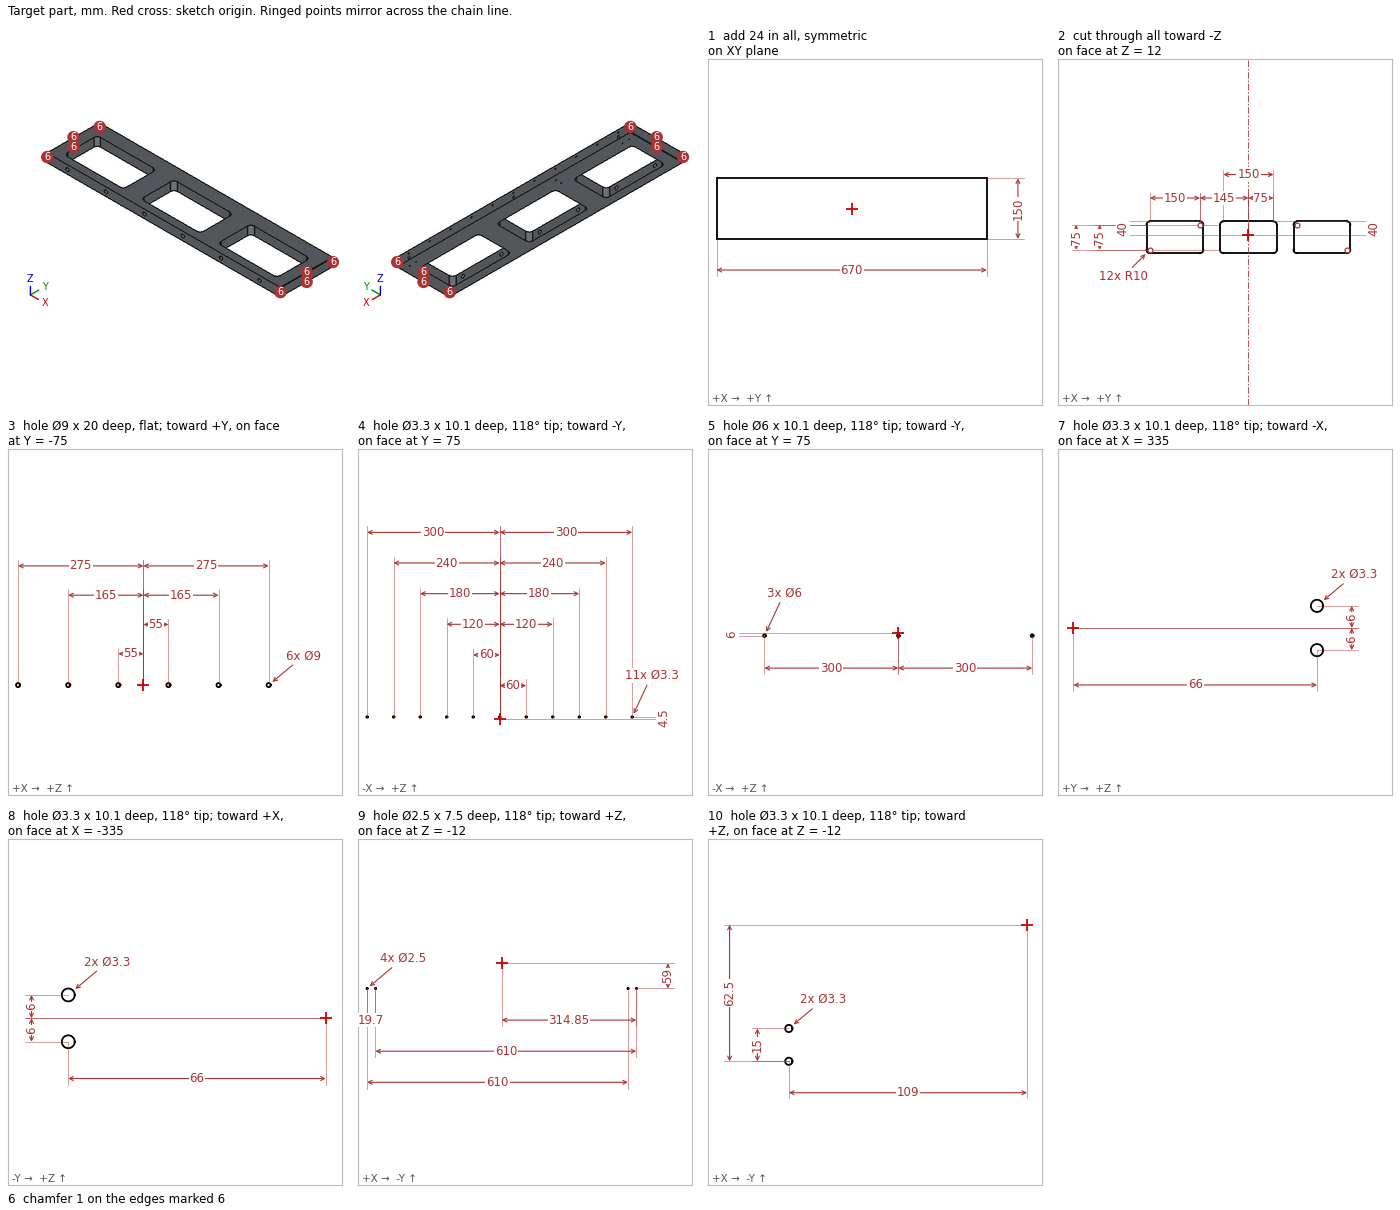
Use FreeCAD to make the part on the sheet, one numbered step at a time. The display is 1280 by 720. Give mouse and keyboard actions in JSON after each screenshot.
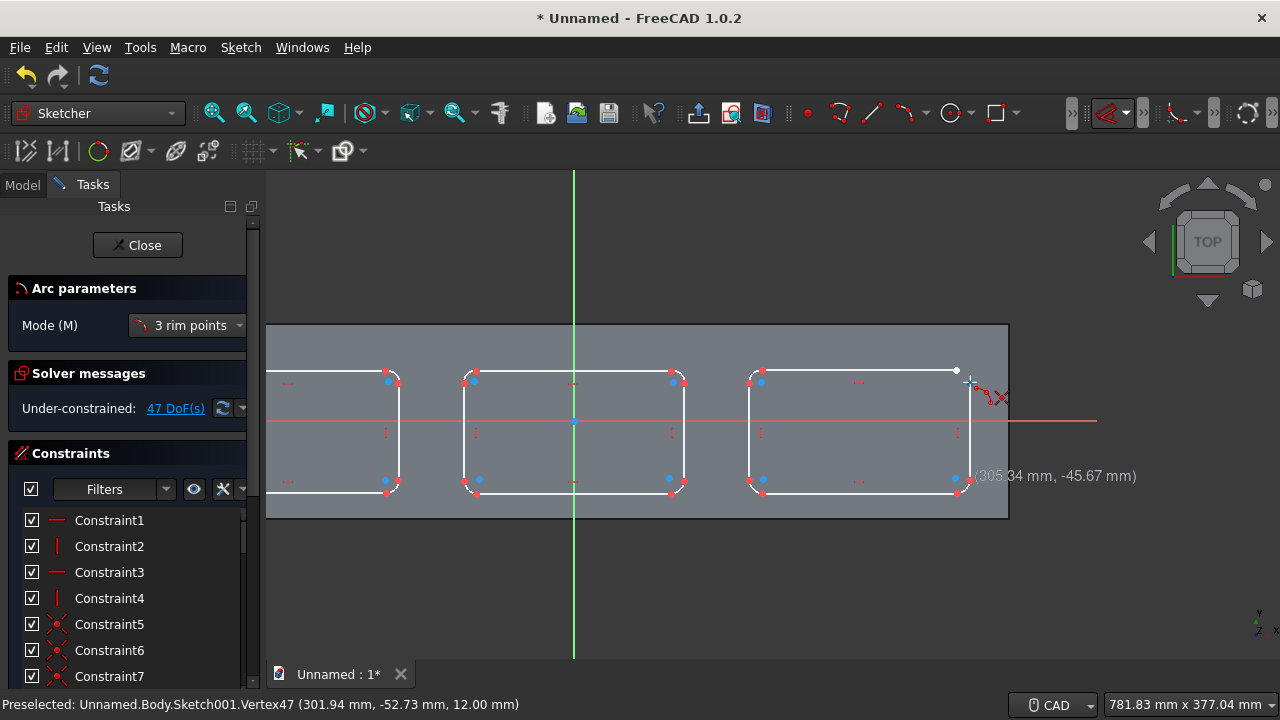
{"action": "left_click", "coordinate": [970, 384]}
{"action": "left_click", "coordinate": [956, 370]}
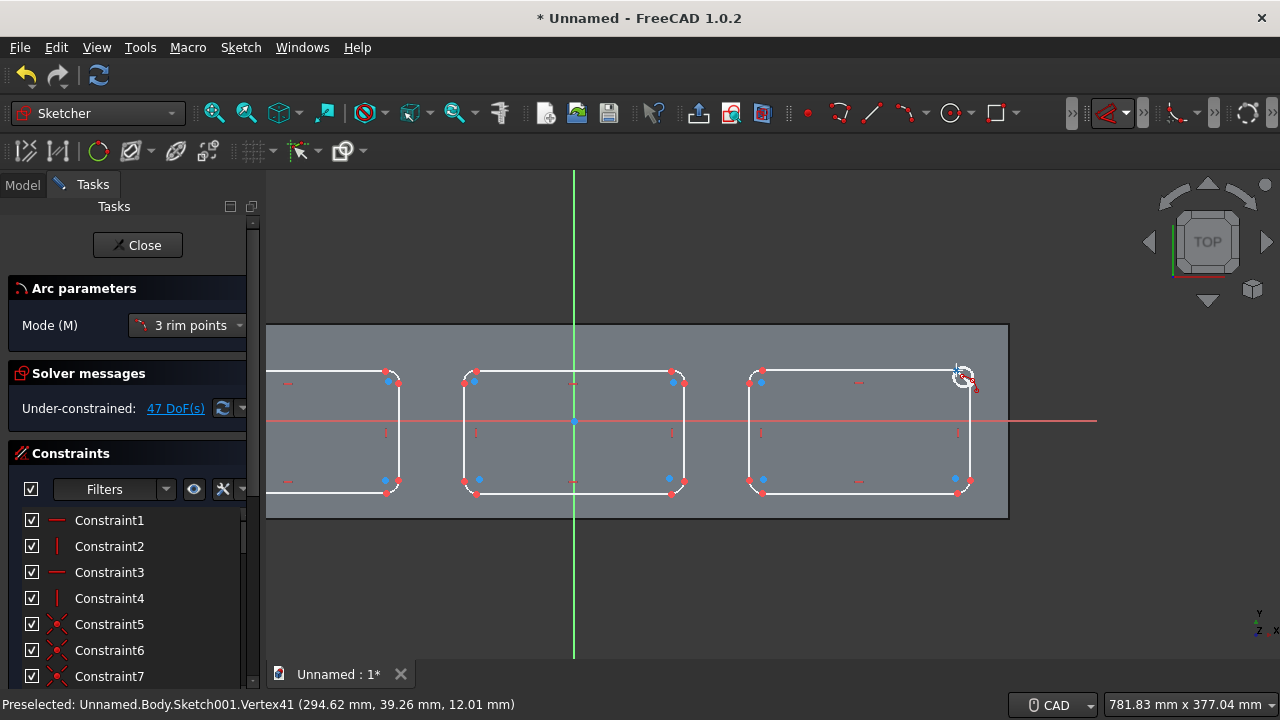
{"action": "scroll", "coordinate": [966, 373], "scroll_direction": "up", "scroll_amount": 8}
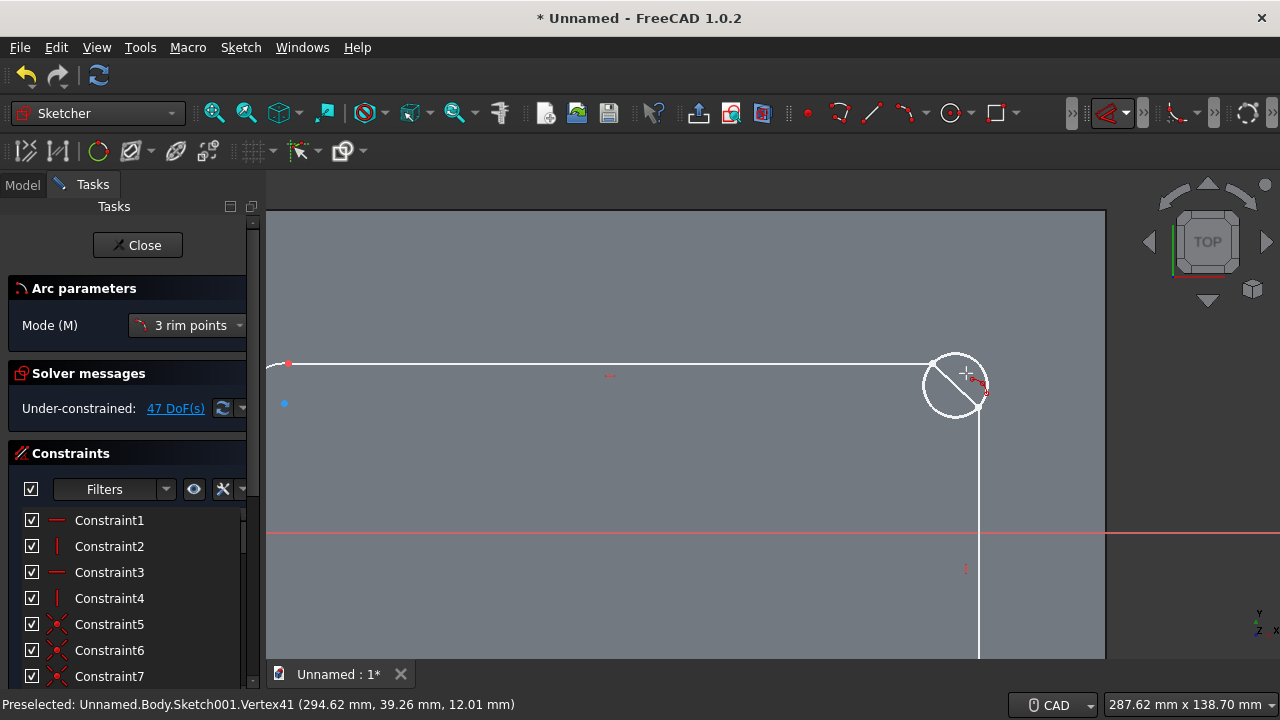
{"action": "left_click", "coordinate": [963, 373]}
{"action": "key", "text": "Escape"}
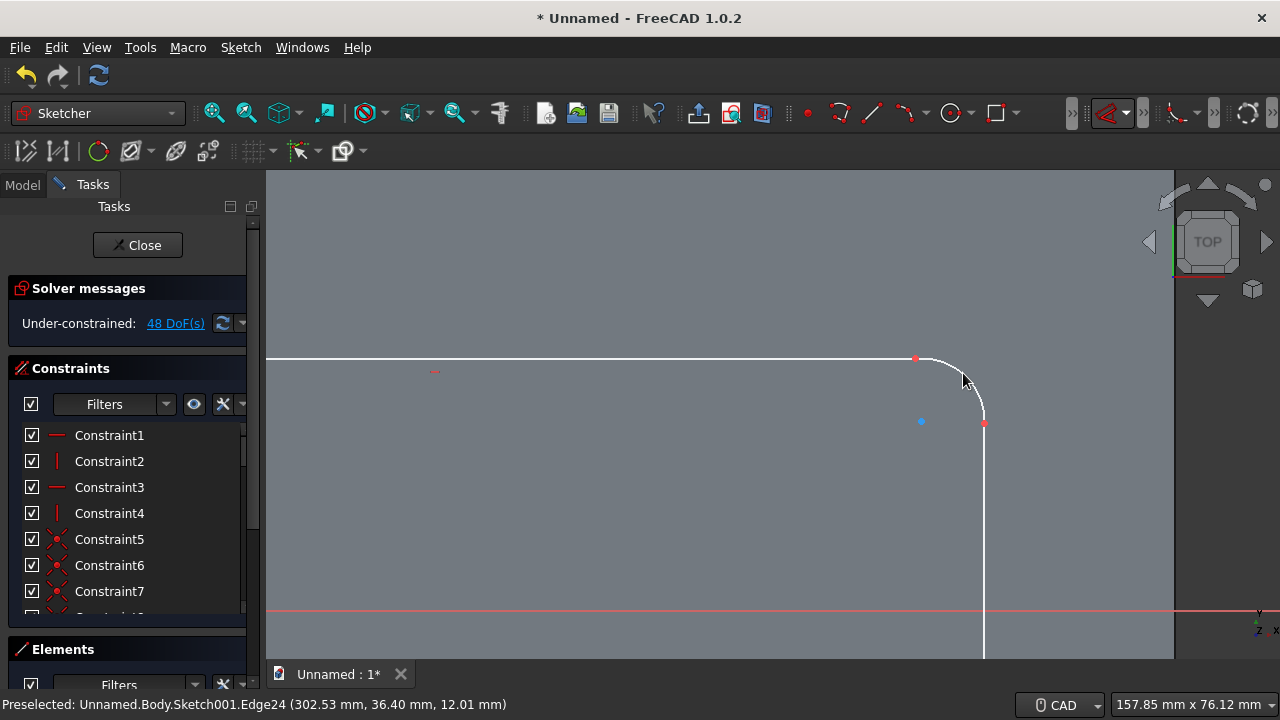
{"action": "scroll", "coordinate": [968, 376], "scroll_direction": "down", "scroll_amount": 10}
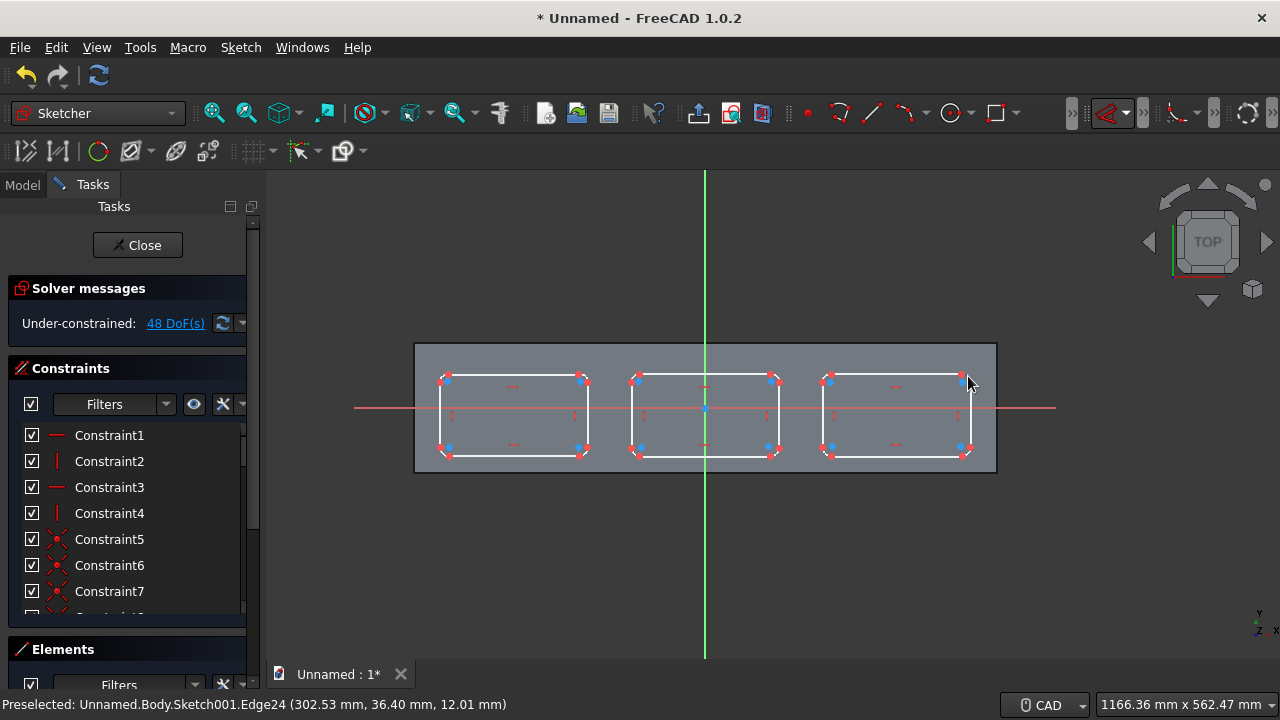
{"action": "left_click", "coordinate": [540, 375]}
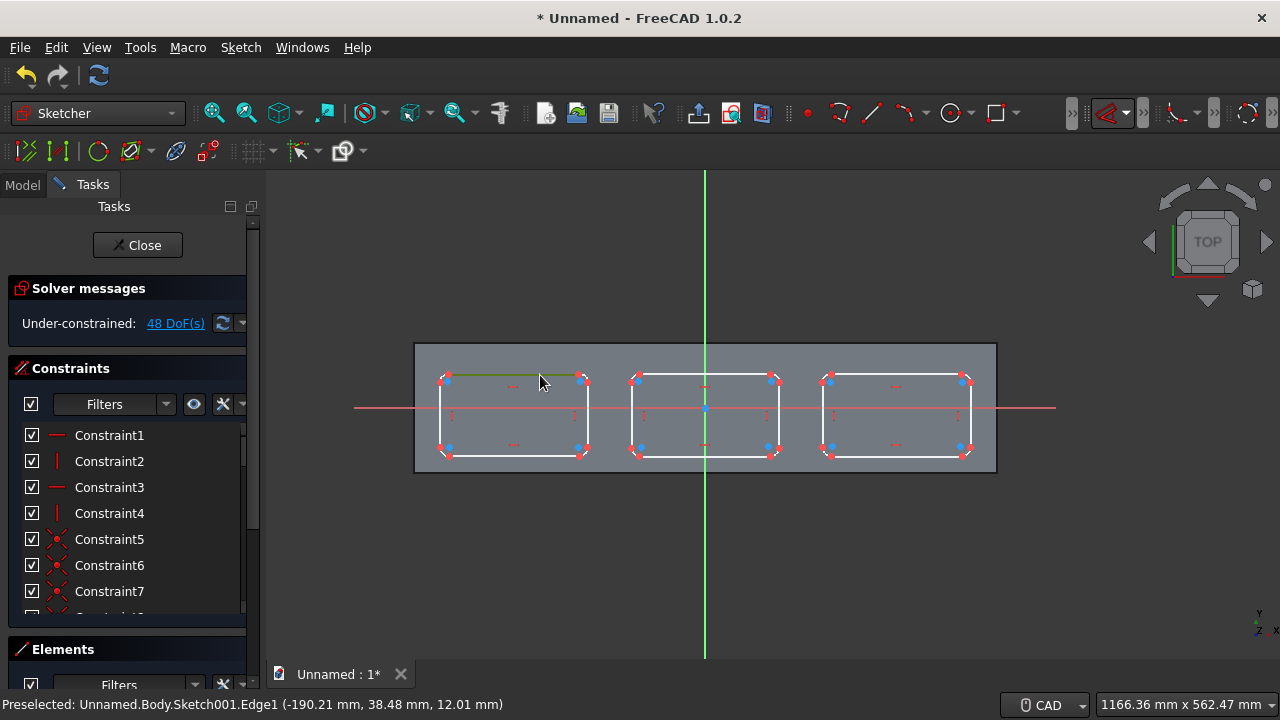
{"action": "scroll", "coordinate": [442, 377], "scroll_direction": "up", "scroll_amount": 4}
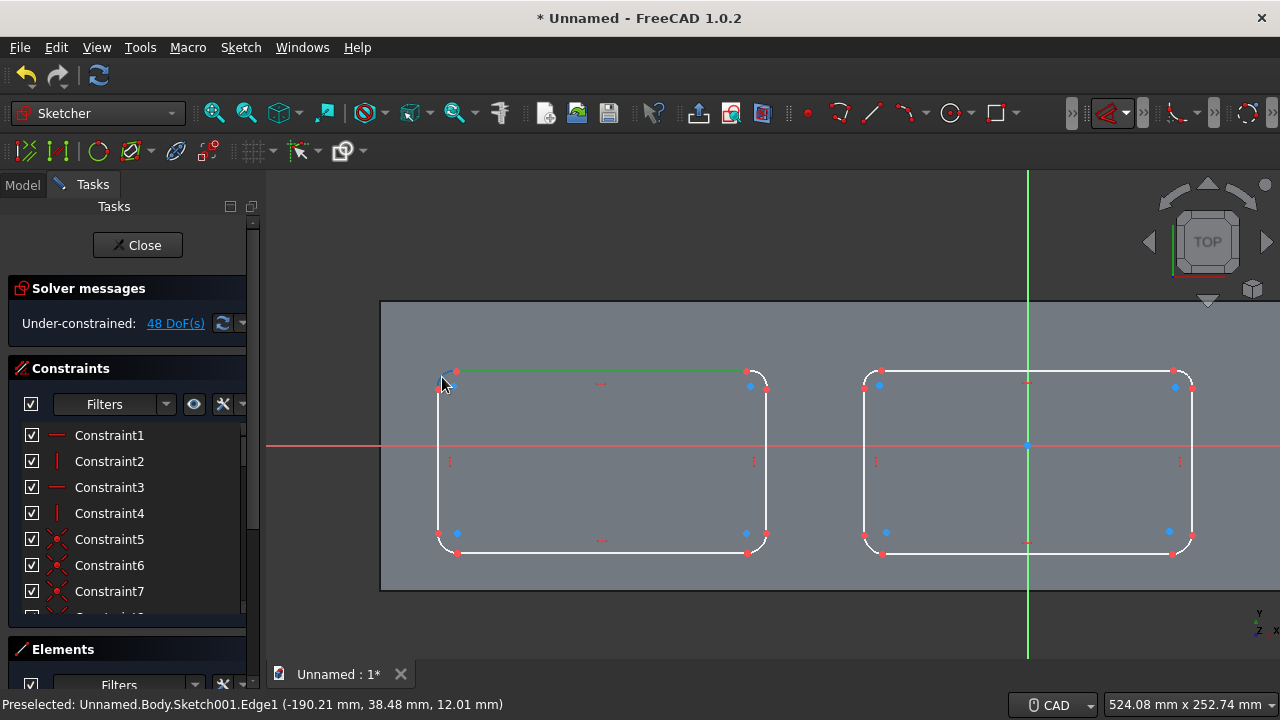
{"action": "left_click", "coordinate": [442, 375]}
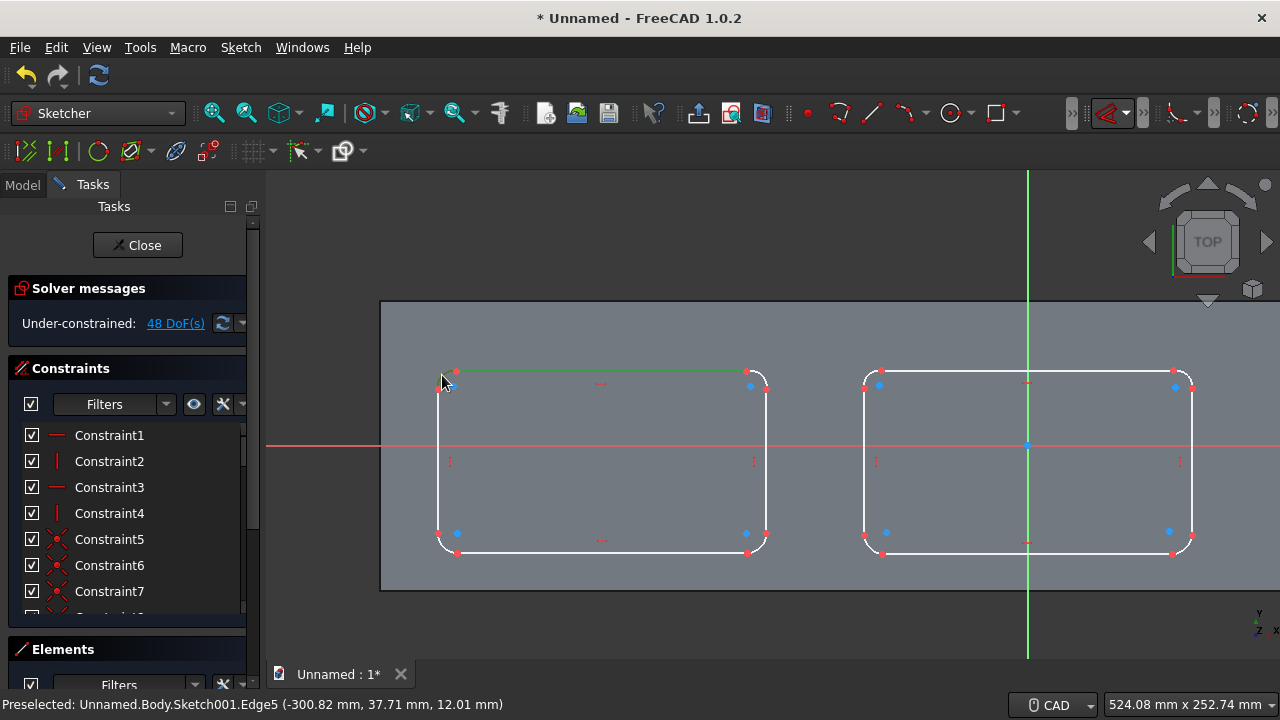
{"action": "key", "text": "t"}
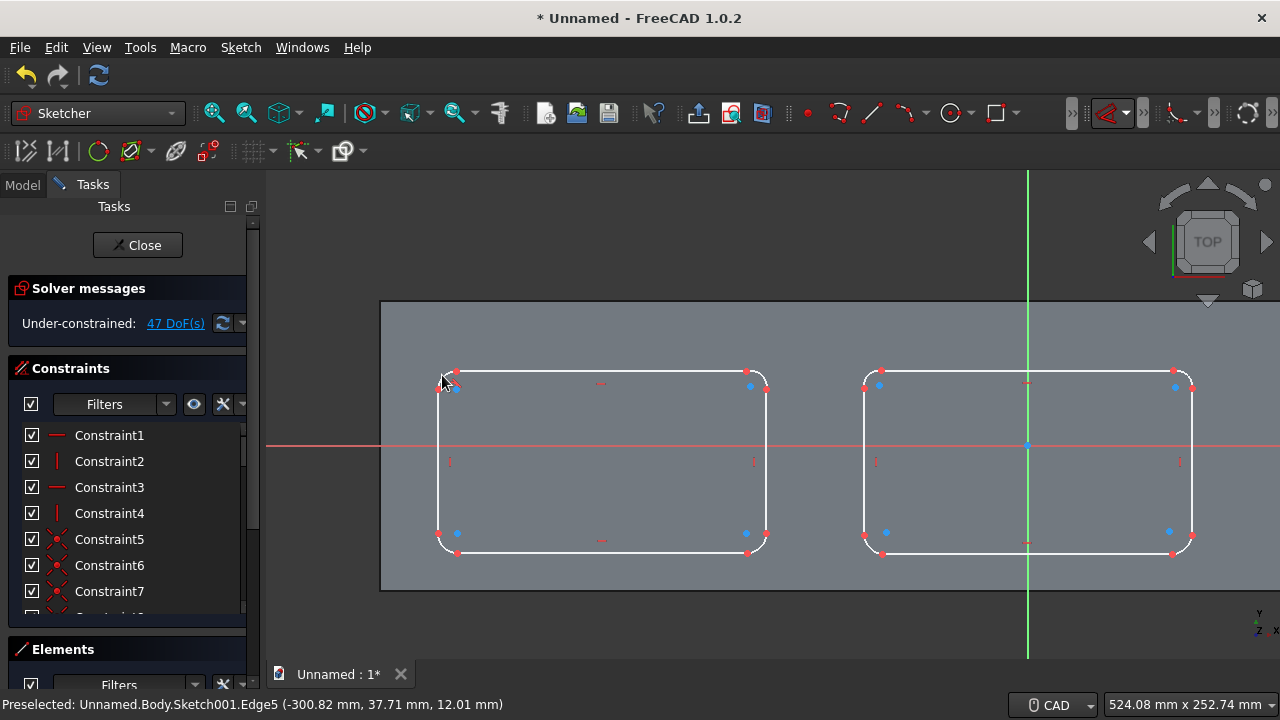
{"action": "left_click", "coordinate": [659, 371]}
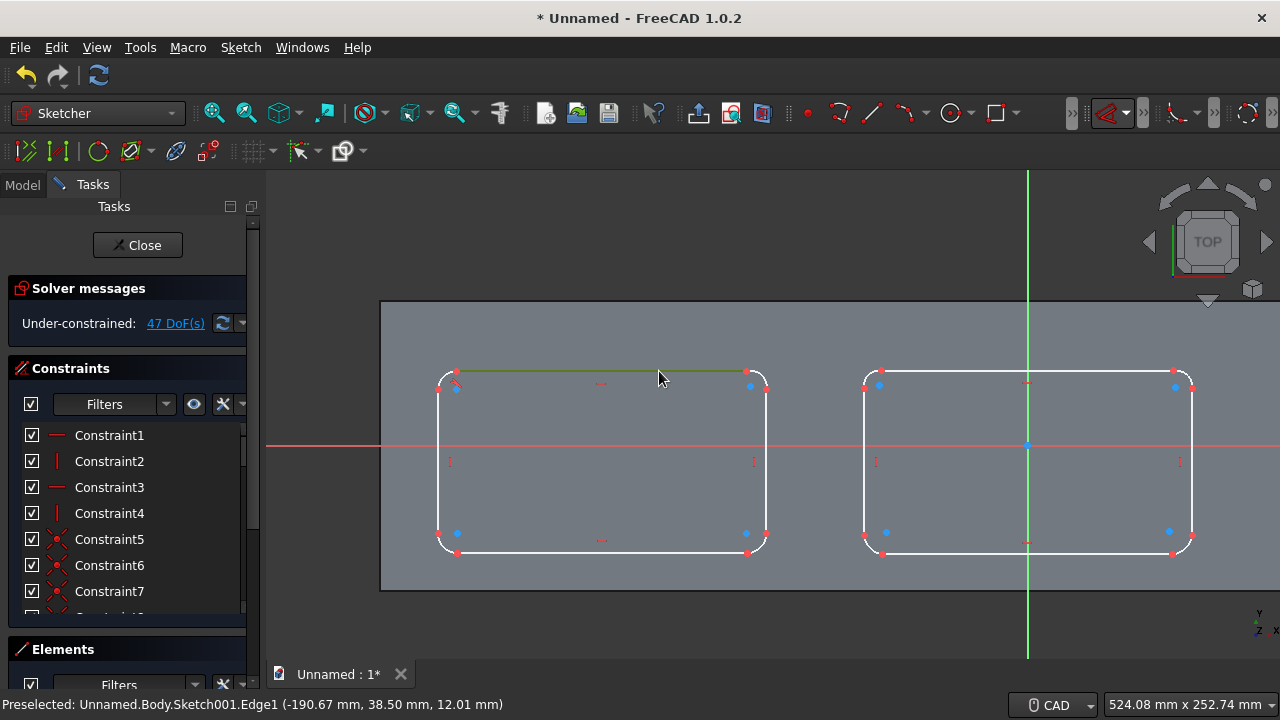
{"action": "scroll", "coordinate": [765, 380], "scroll_direction": "up", "scroll_amount": 2}